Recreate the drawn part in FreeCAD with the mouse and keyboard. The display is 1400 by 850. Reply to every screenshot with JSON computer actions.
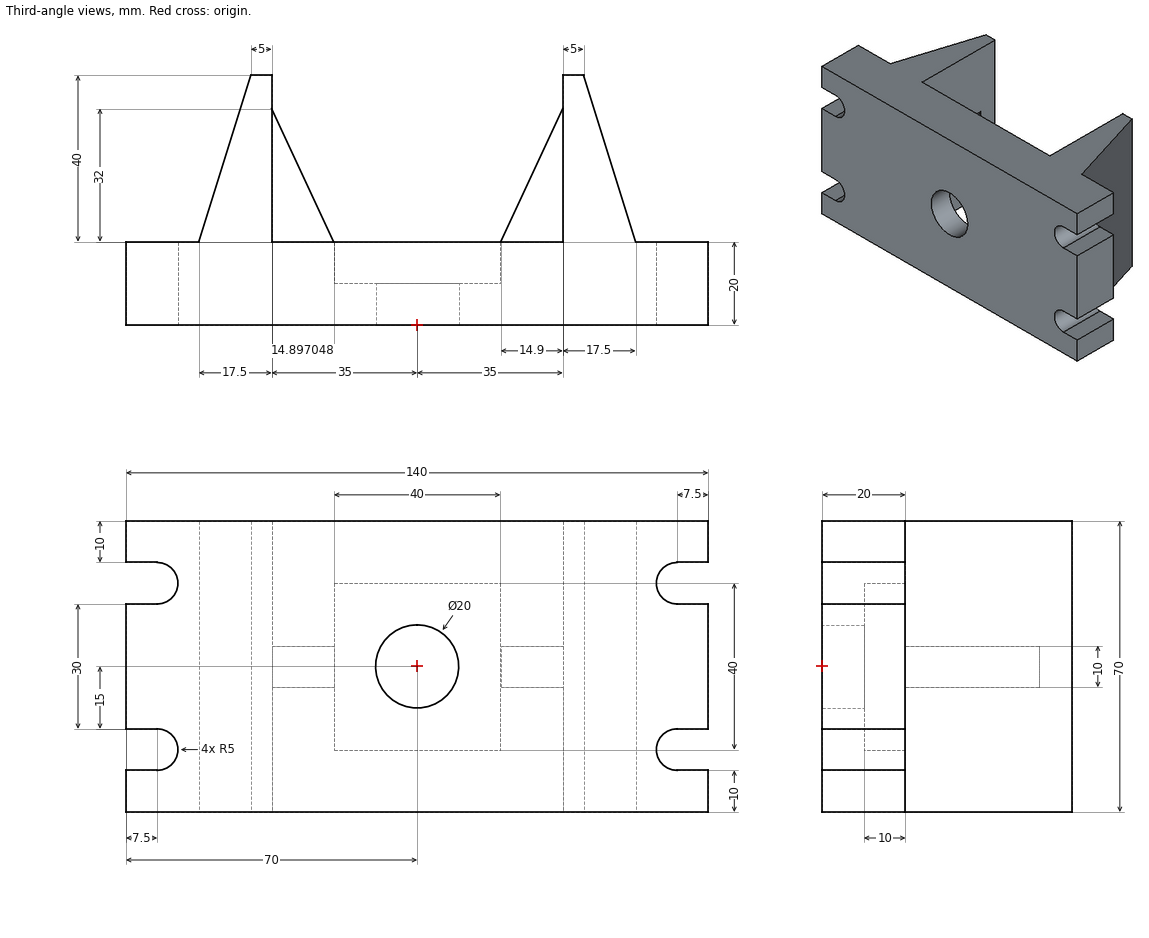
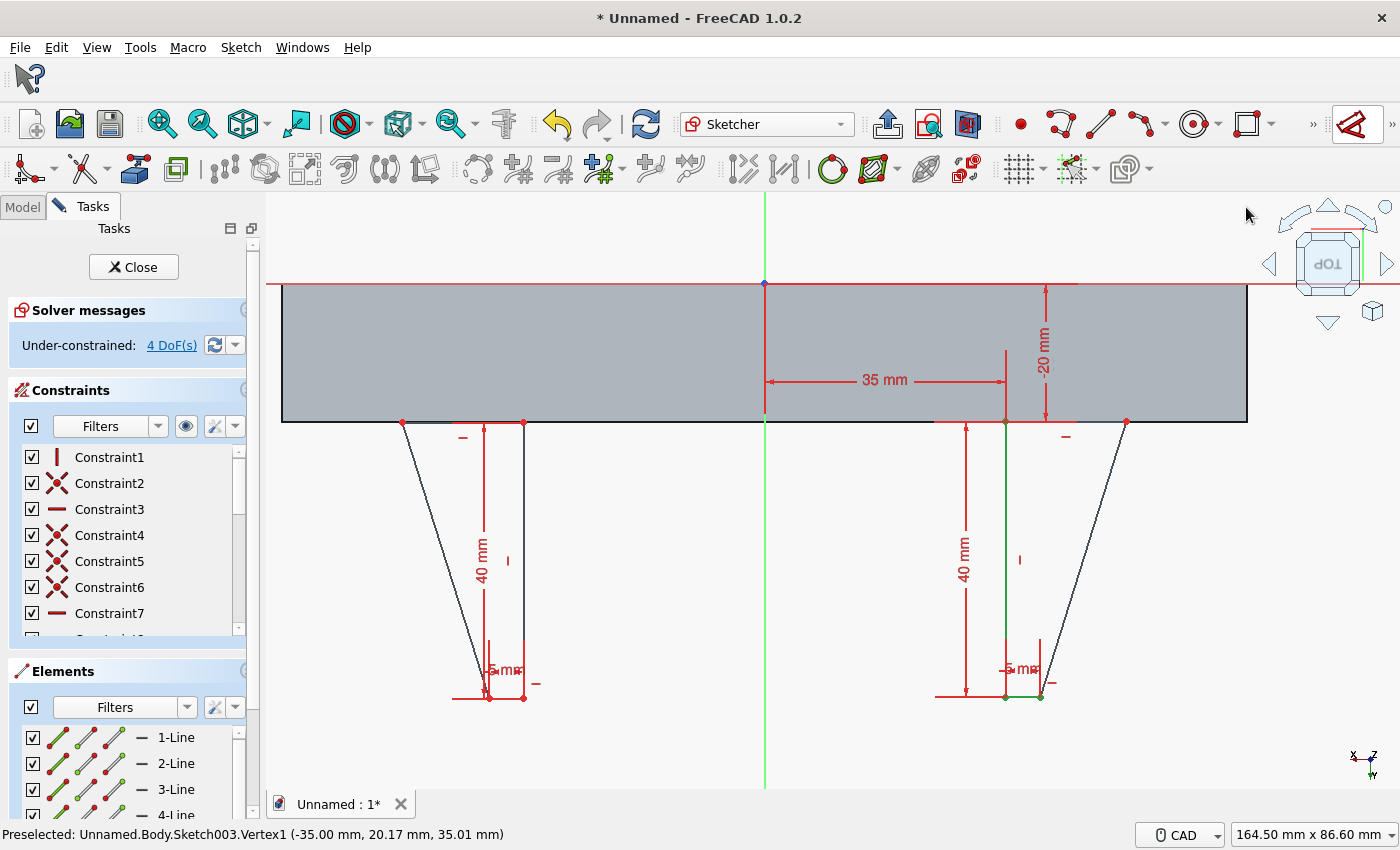
{"action": "left_click", "coordinate": [524, 423]}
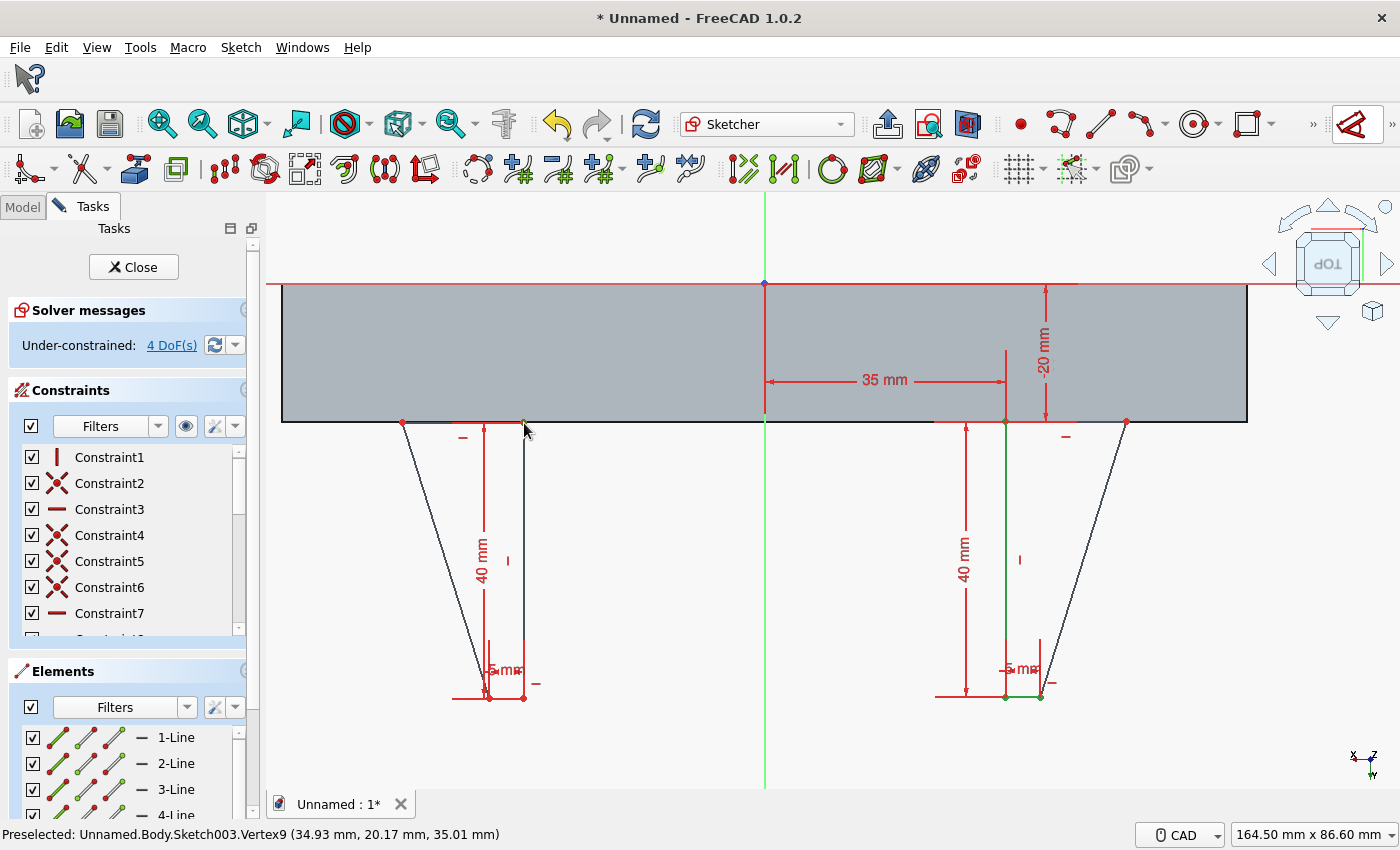
{"action": "left_click", "coordinate": [1378, 124]}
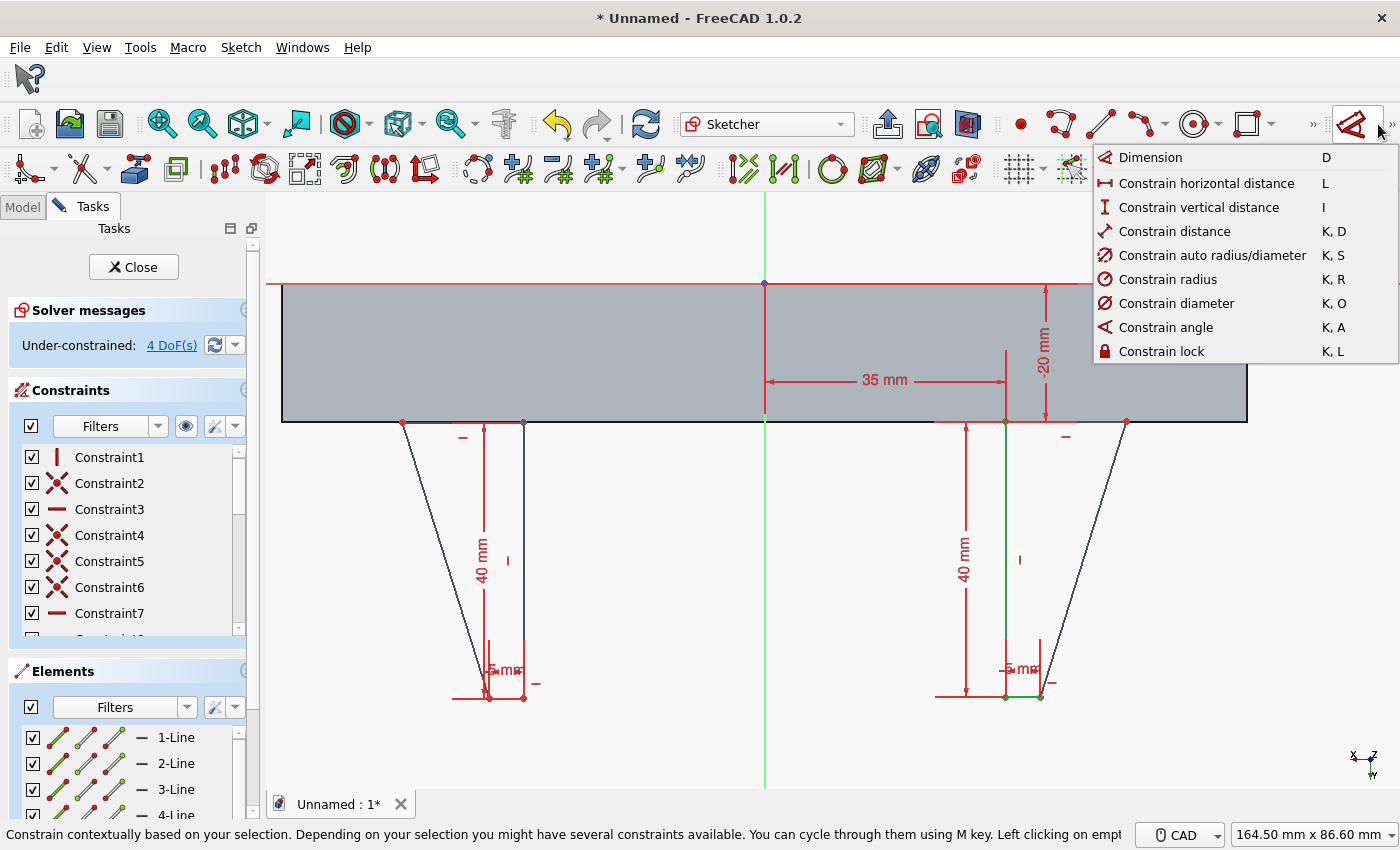
{"action": "left_click", "coordinate": [1246, 183]}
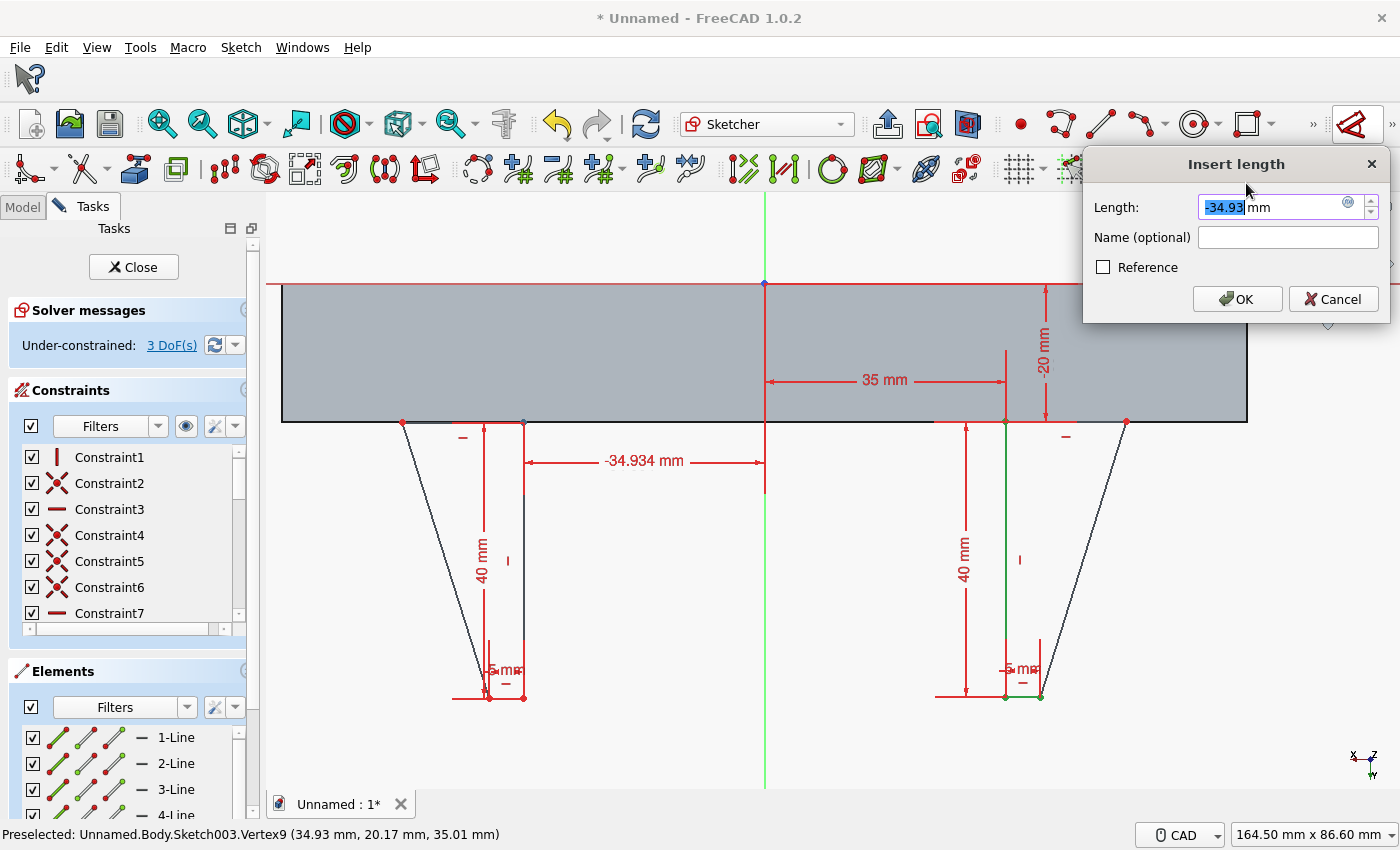
{"action": "type", "text": "-35"}
{"action": "key", "text": "Return"}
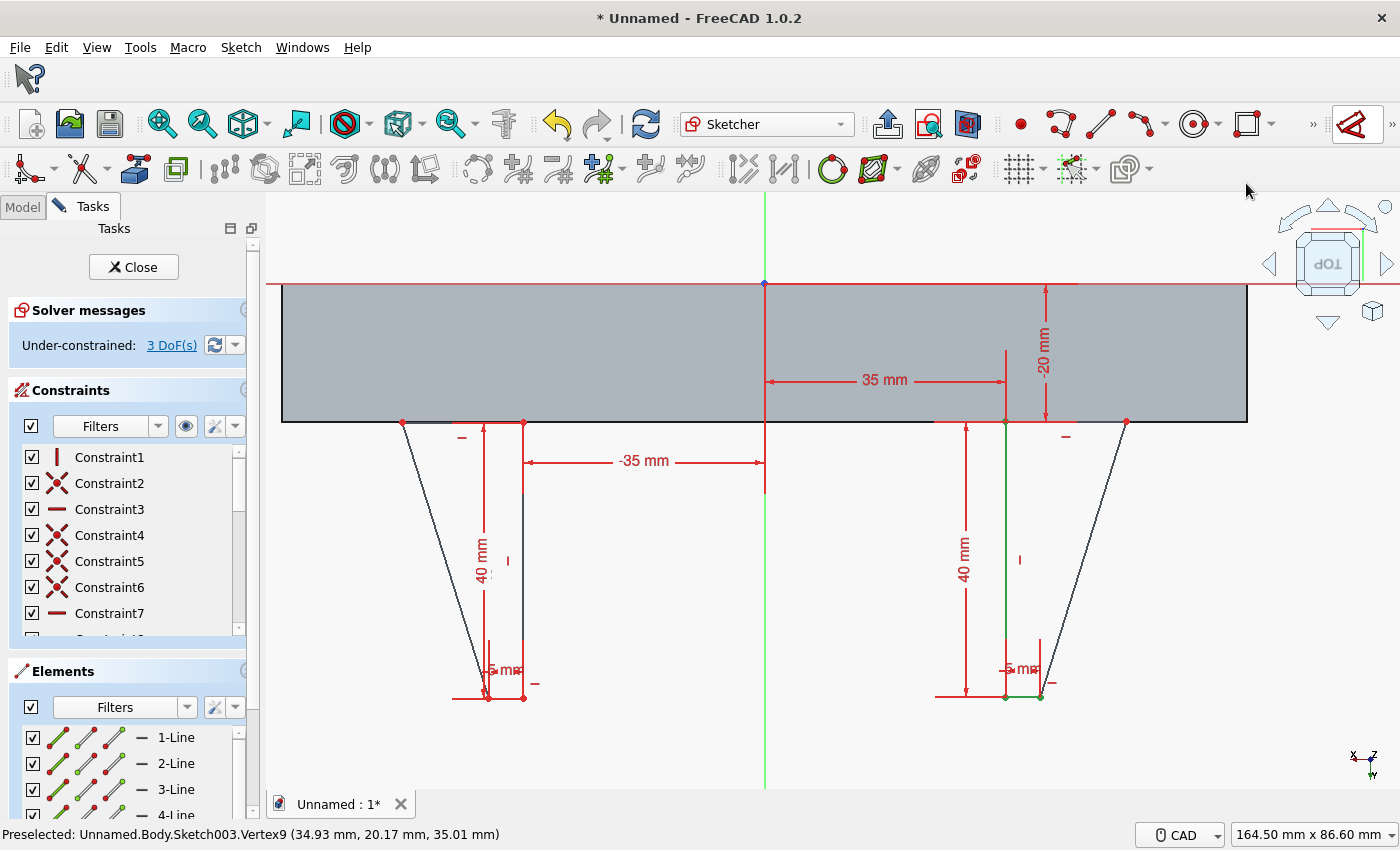
{"action": "left_click", "coordinate": [523, 423]}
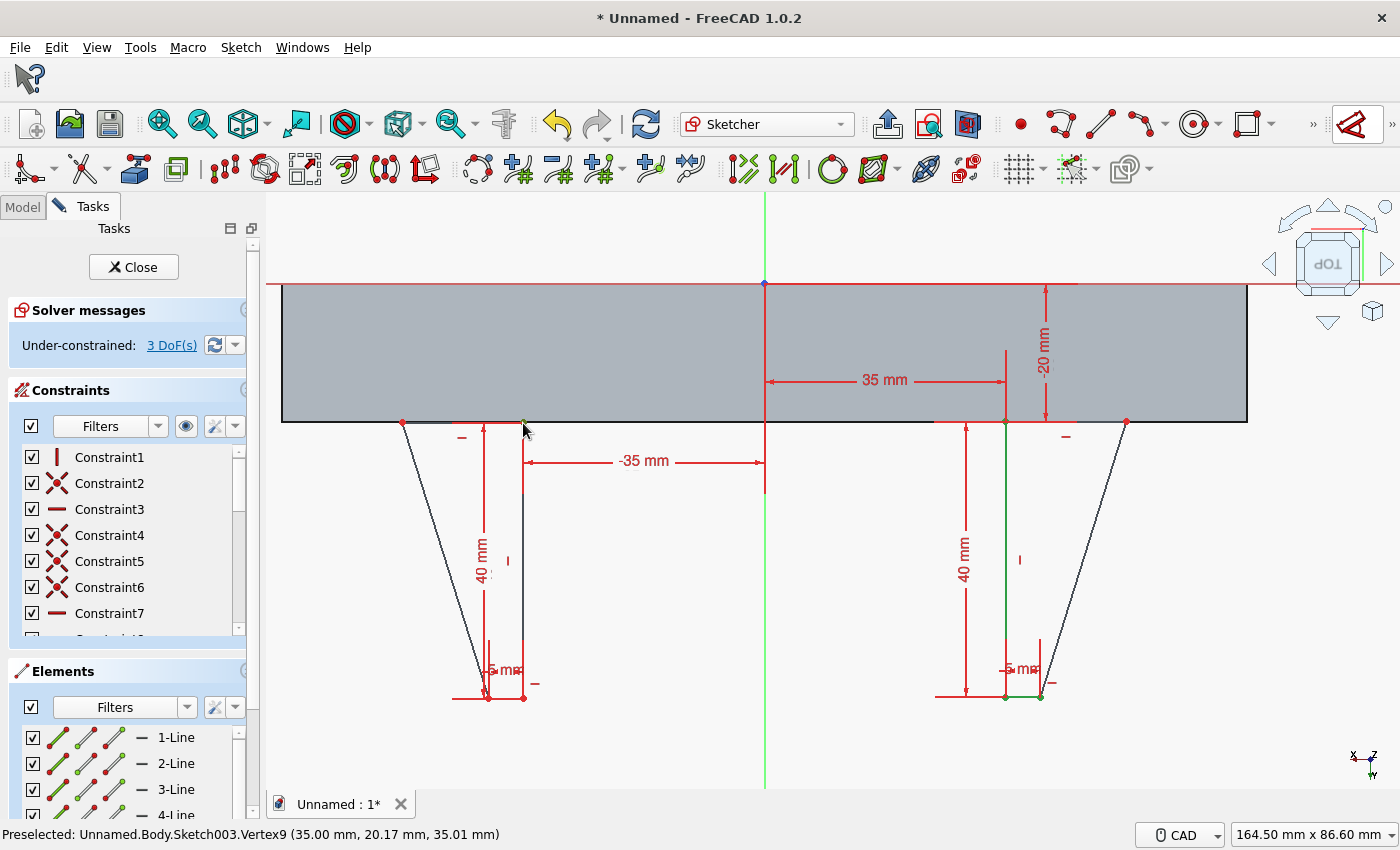
{"action": "left_click", "coordinate": [1378, 124]}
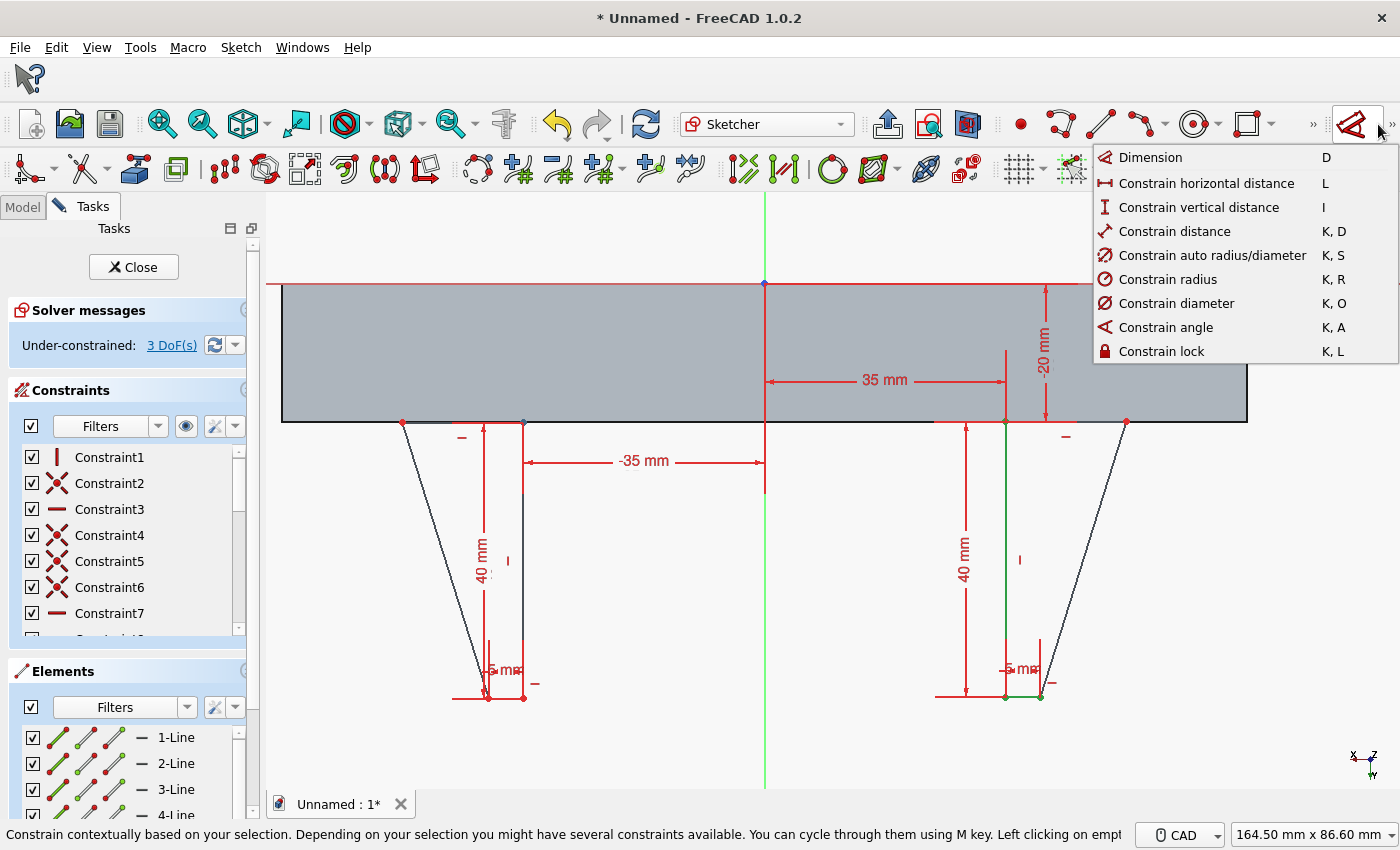
{"action": "left_click", "coordinate": [1246, 207]}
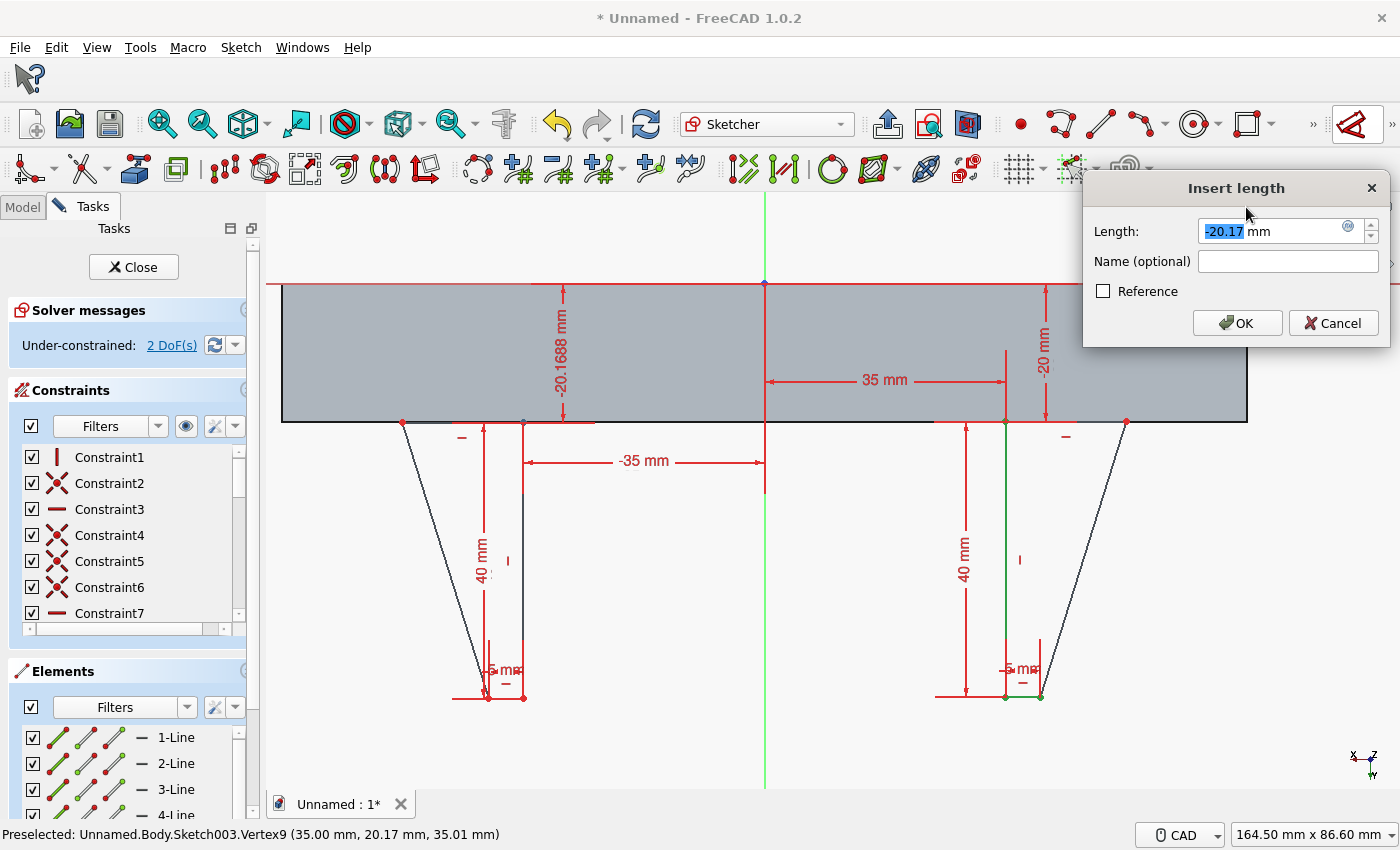
{"action": "type", "text": "-20"}
{"action": "key", "text": "Return"}